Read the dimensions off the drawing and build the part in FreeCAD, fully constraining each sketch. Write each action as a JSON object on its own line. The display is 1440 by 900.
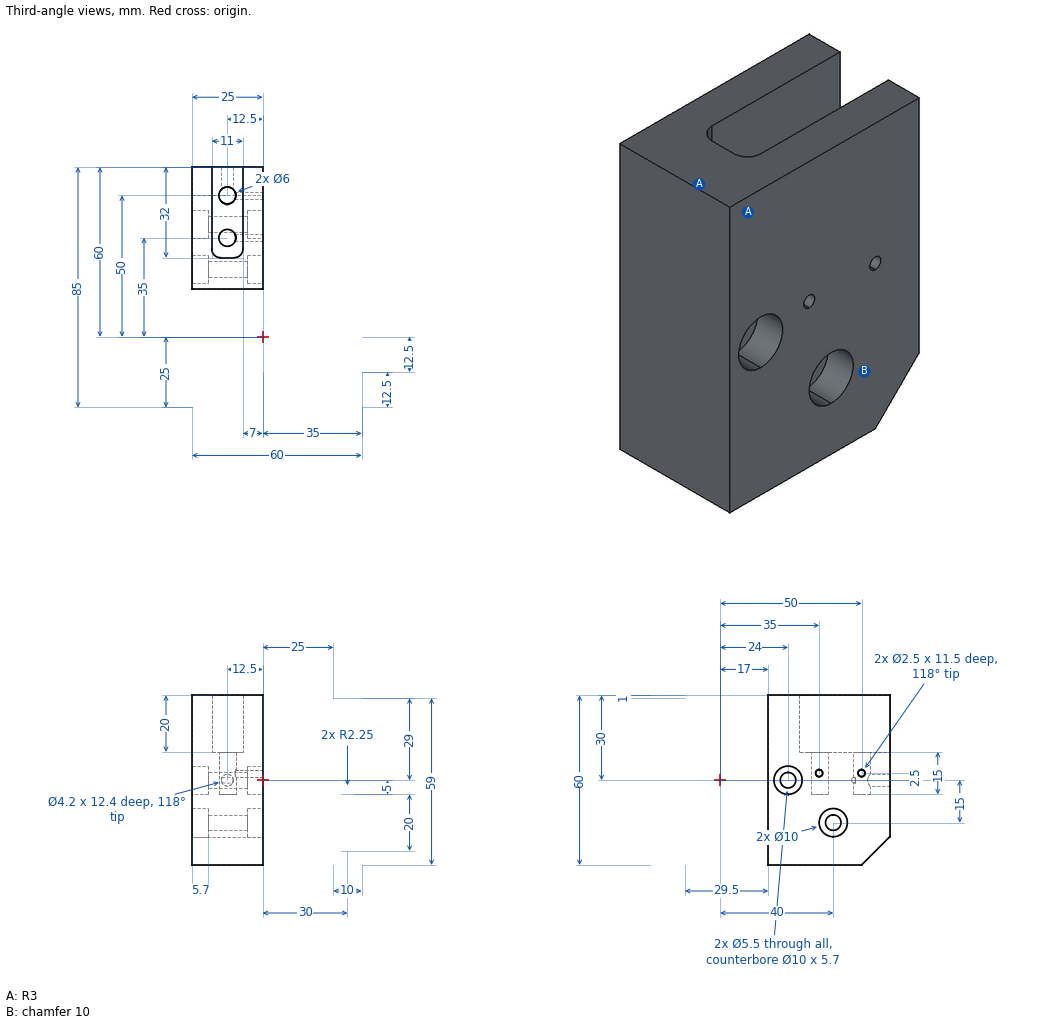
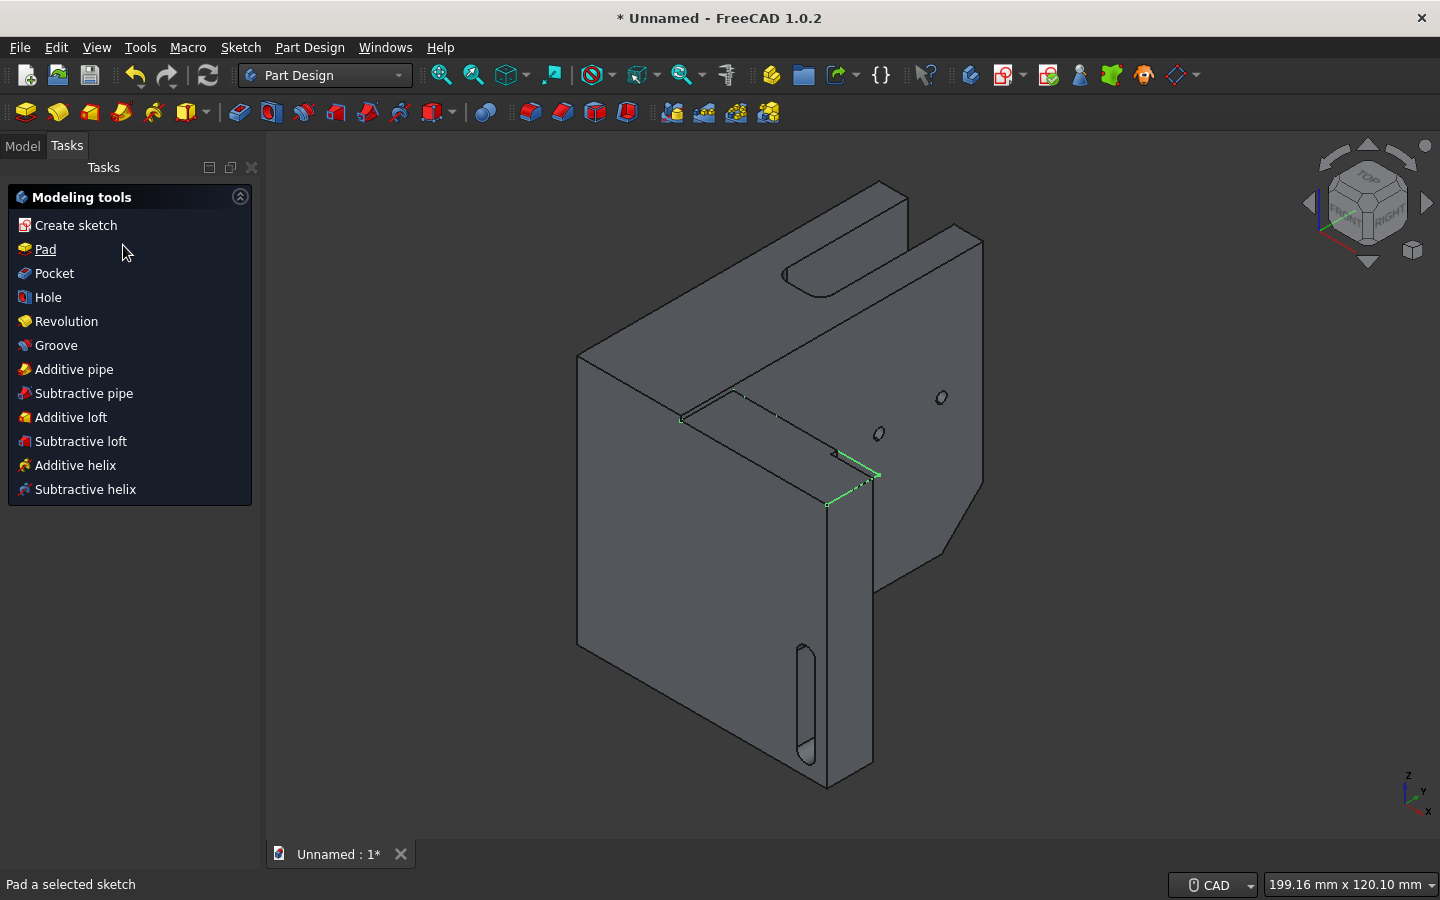
{"action": "left_click", "coordinate": [240, 112]}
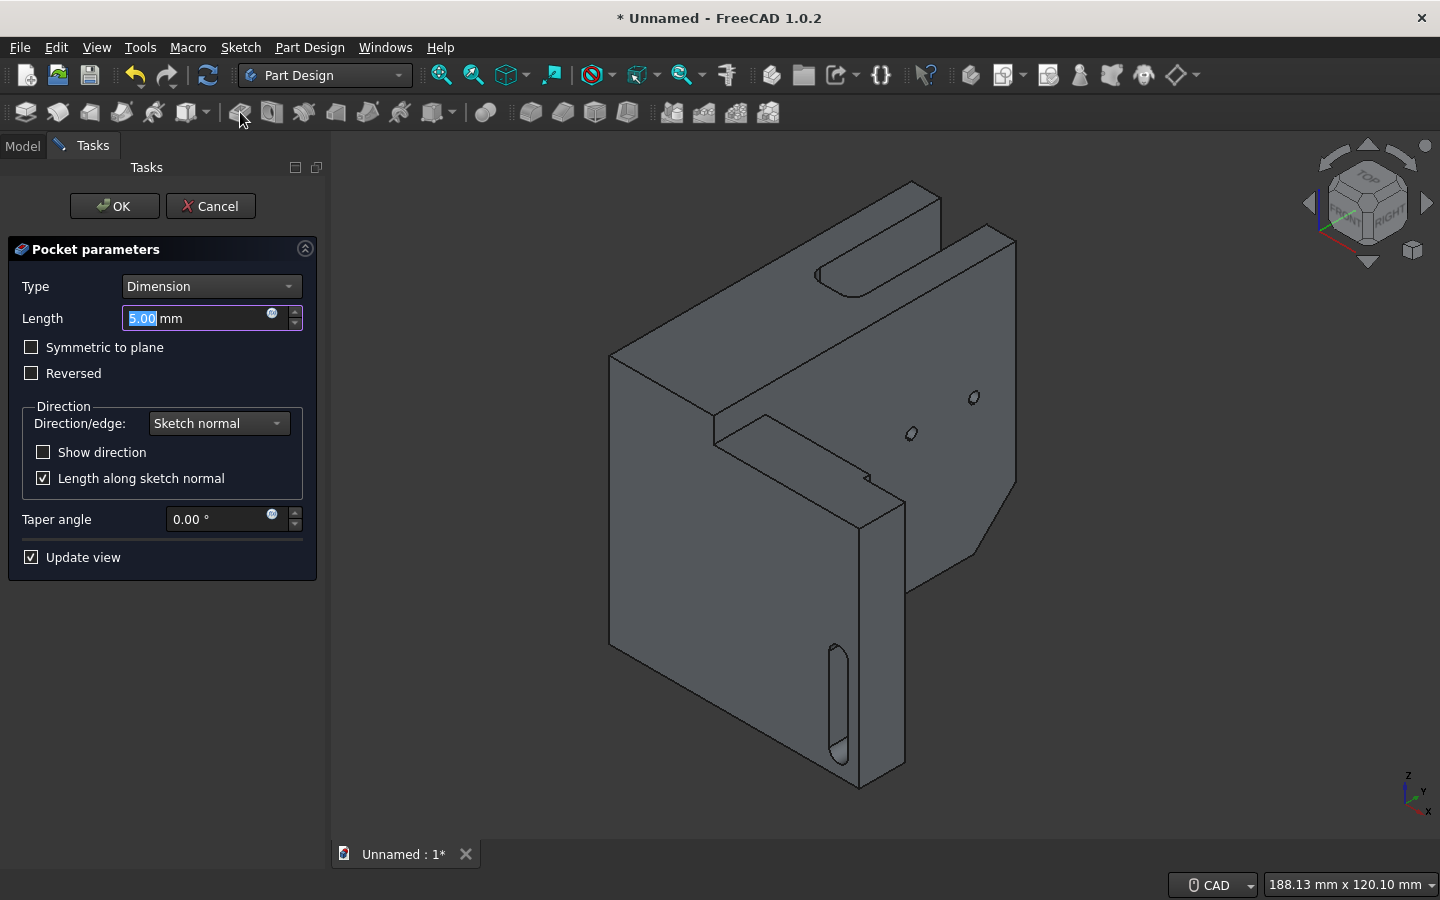
{"action": "left_click", "coordinate": [212, 286]}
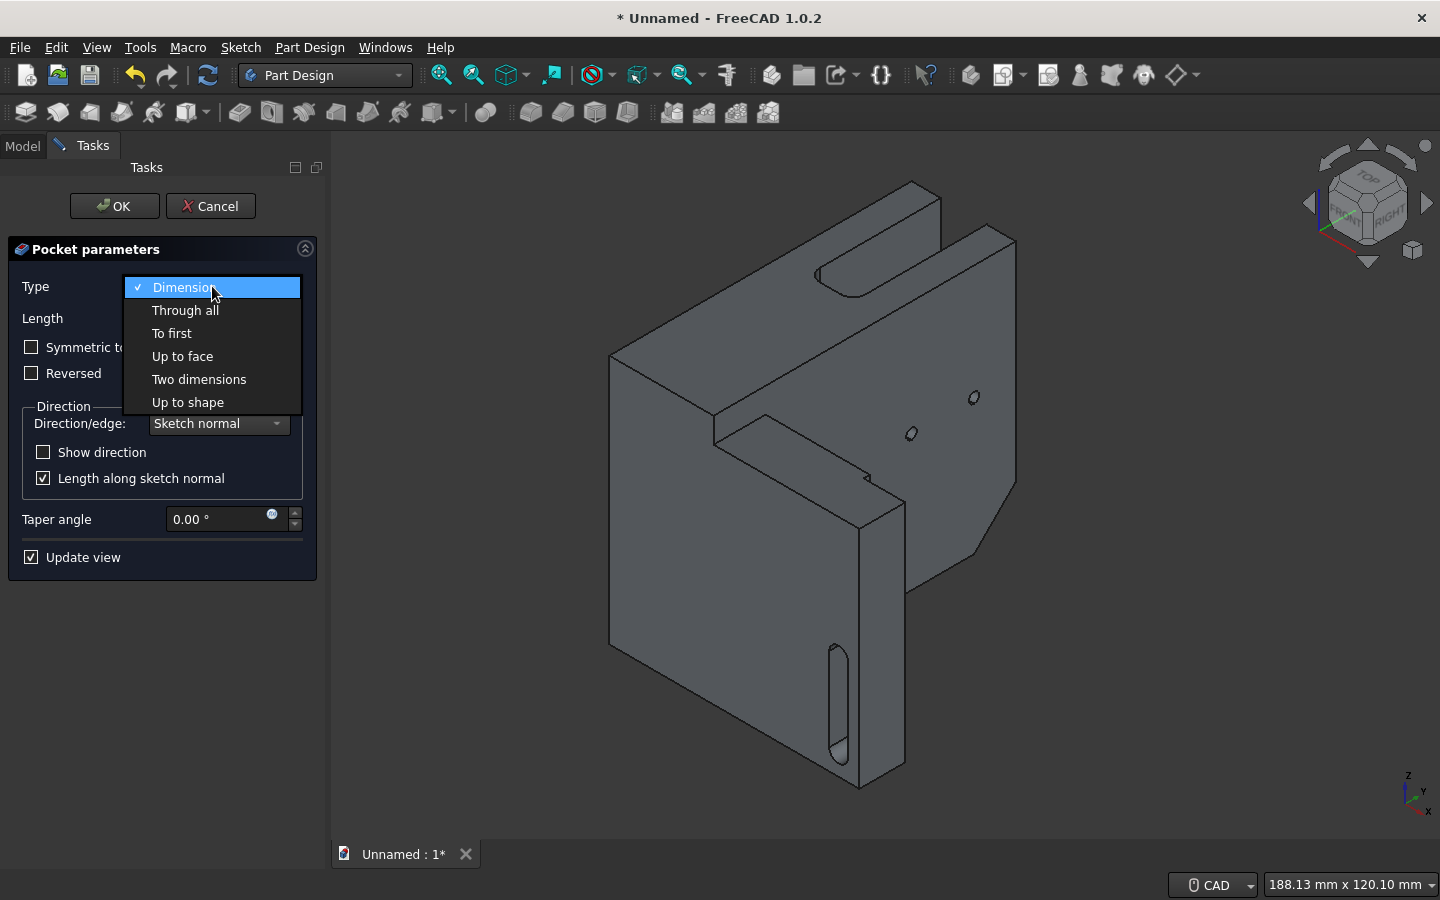
{"action": "left_click", "coordinate": [212, 310]}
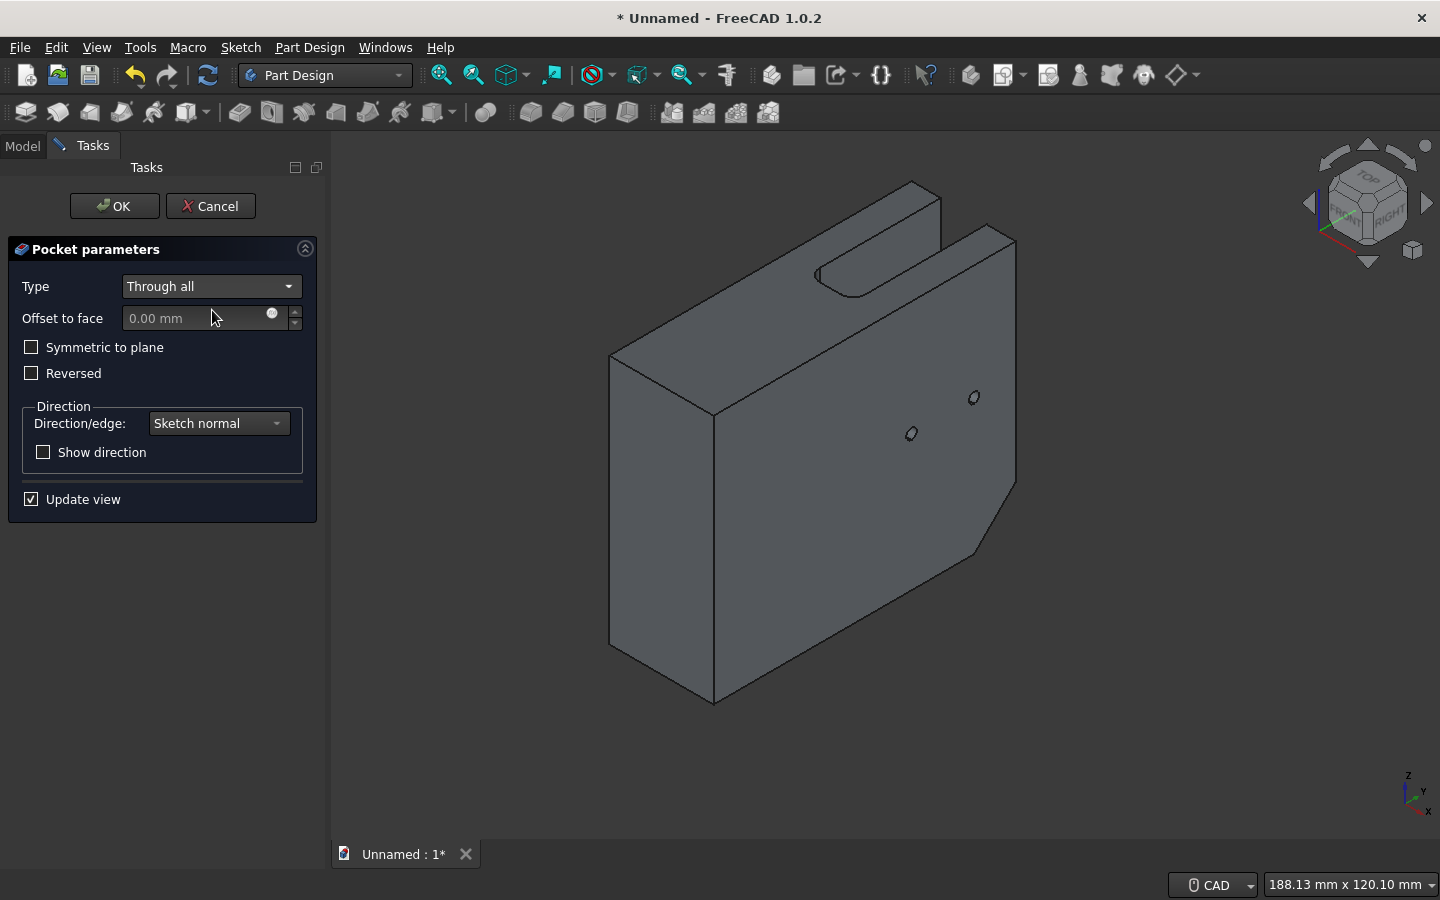
{"action": "left_click", "coordinate": [115, 206]}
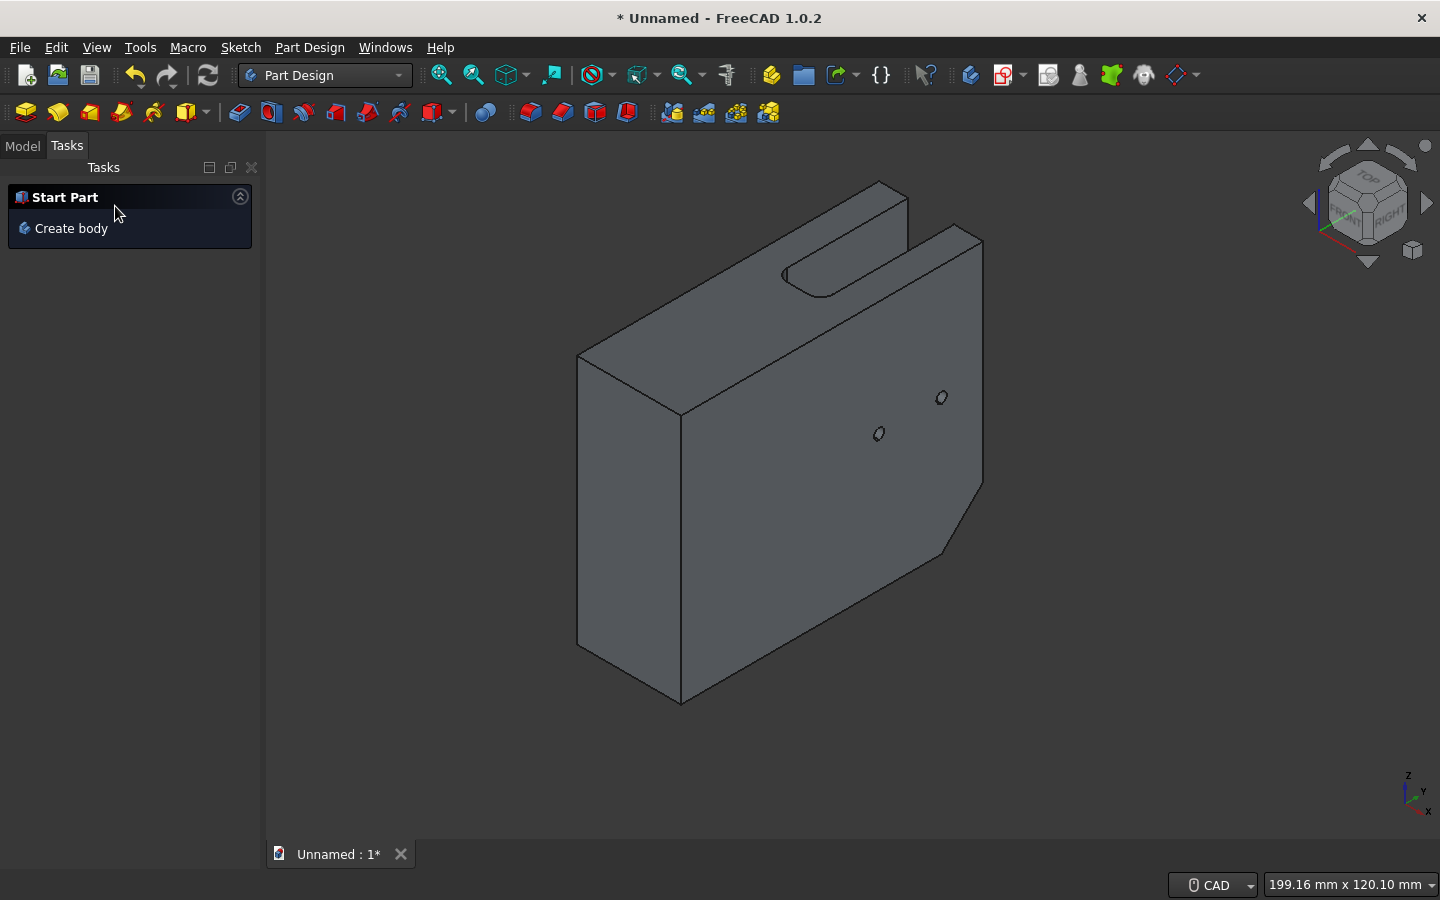
{"action": "left_click", "coordinate": [789, 538]}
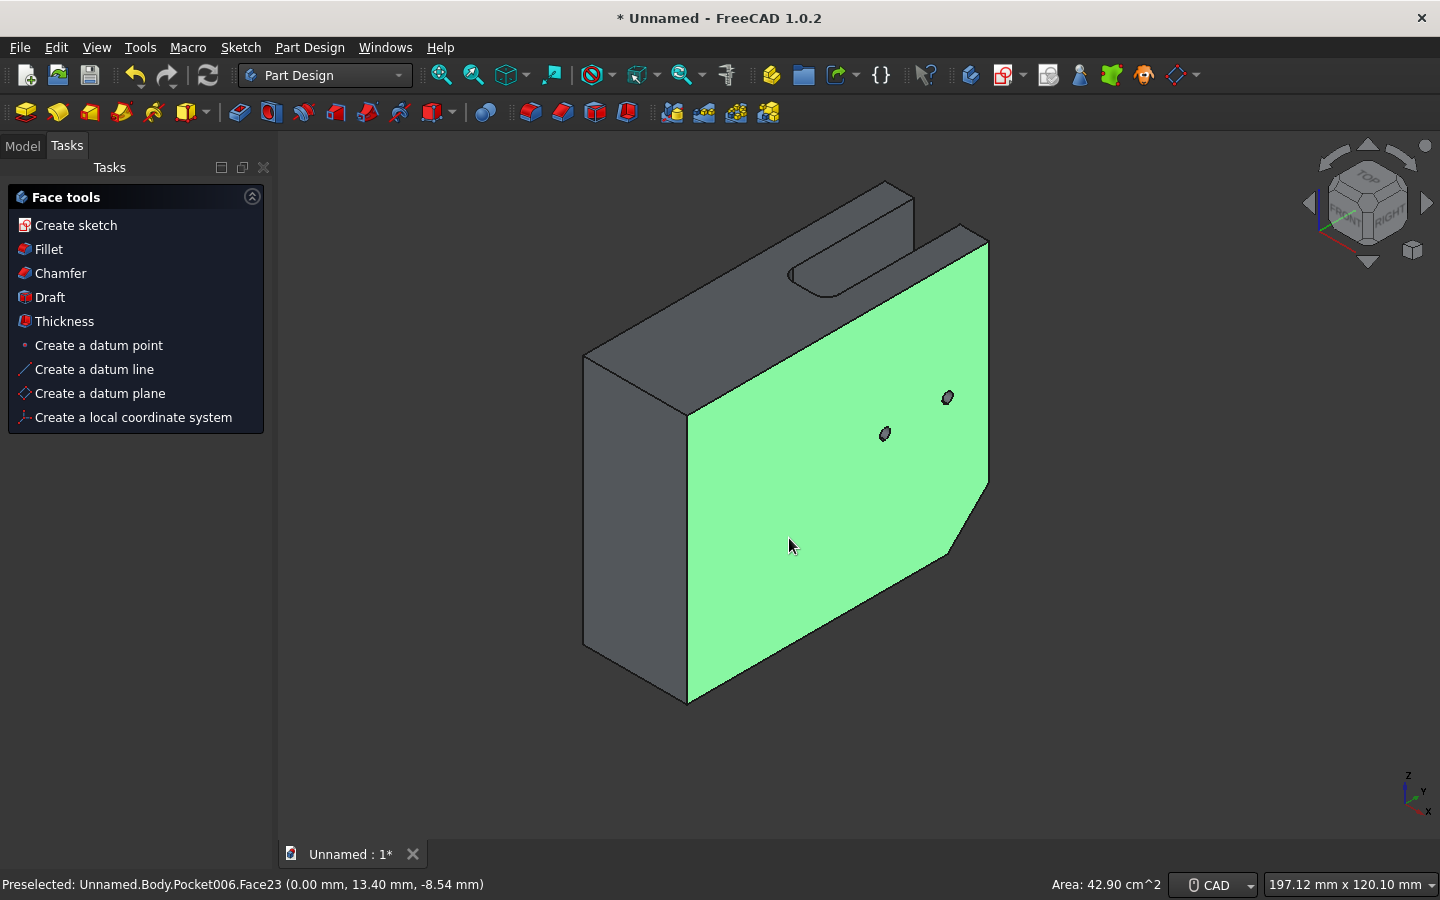
{"action": "left_click", "coordinate": [1004, 76]}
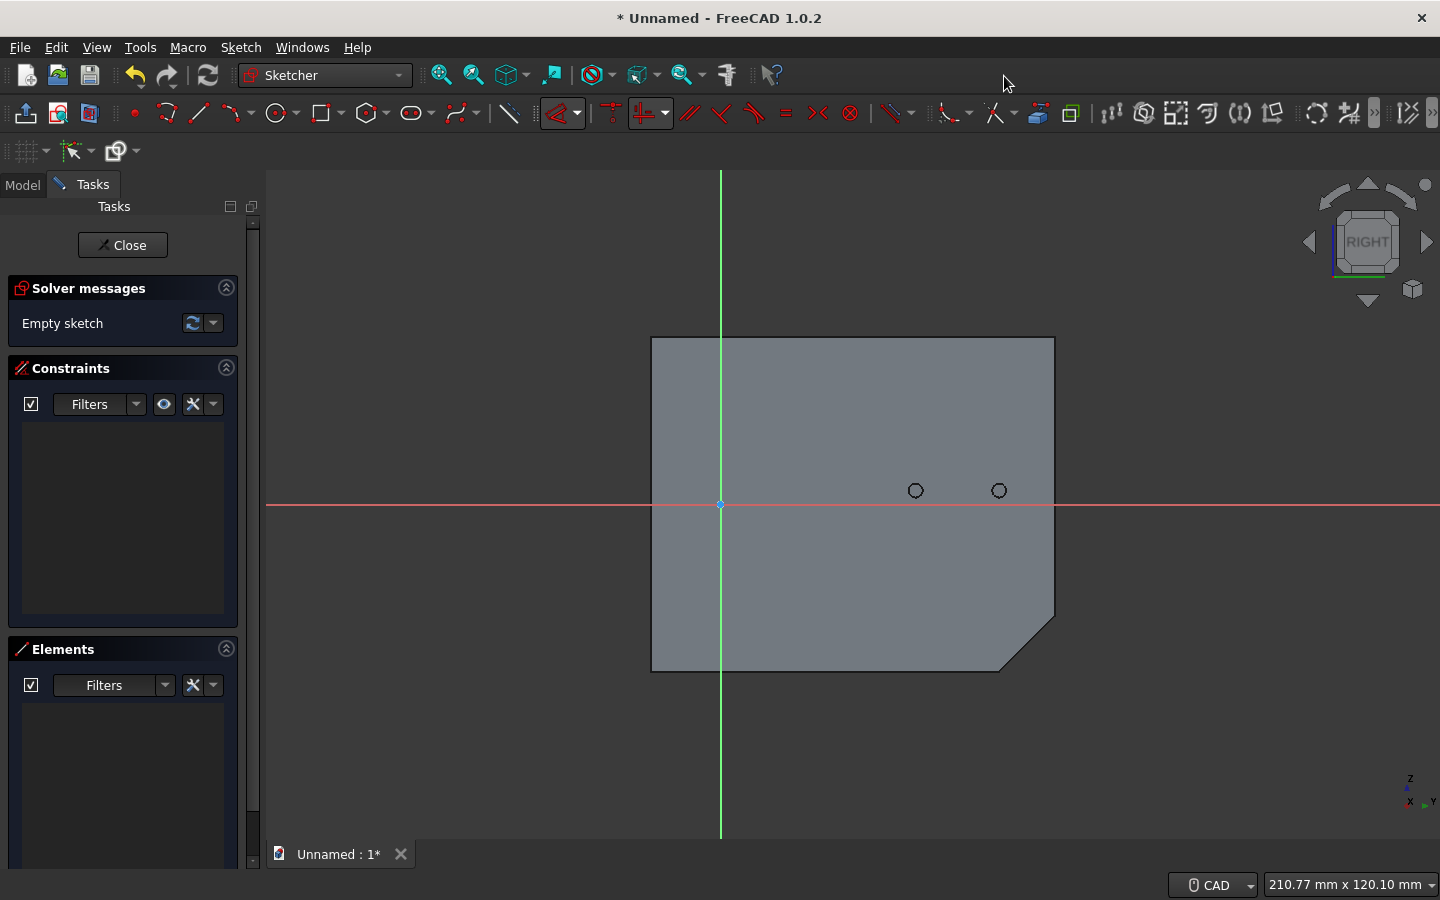
{"action": "scroll", "coordinate": [872, 571], "scroll_direction": "up", "scroll_amount": 5}